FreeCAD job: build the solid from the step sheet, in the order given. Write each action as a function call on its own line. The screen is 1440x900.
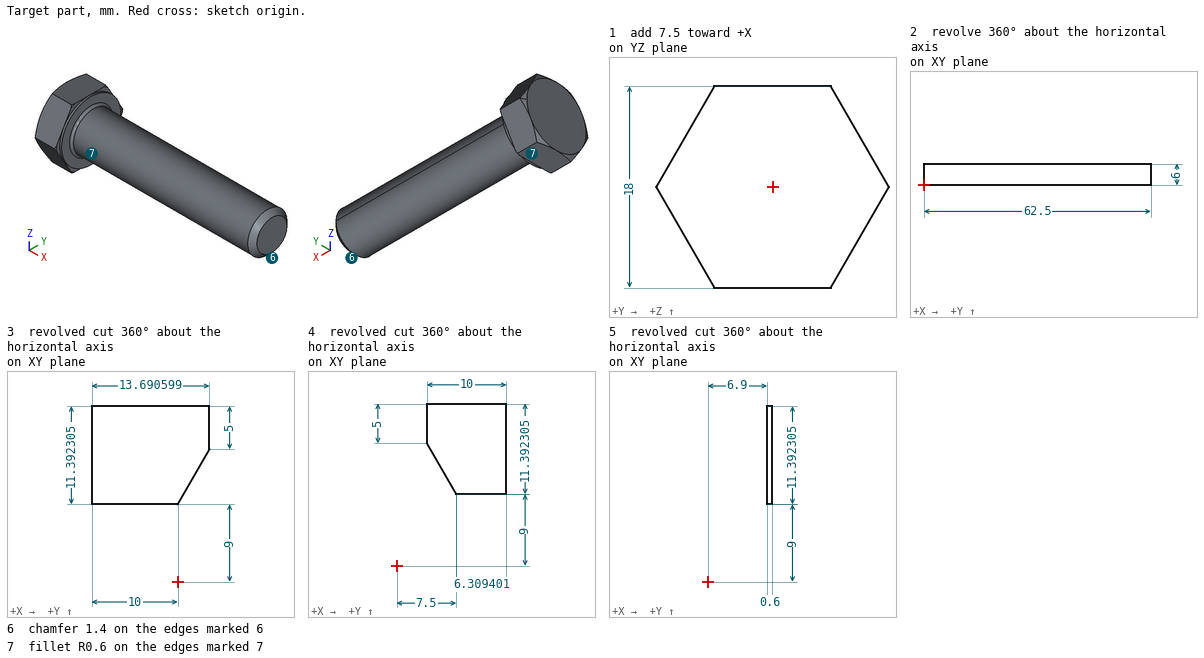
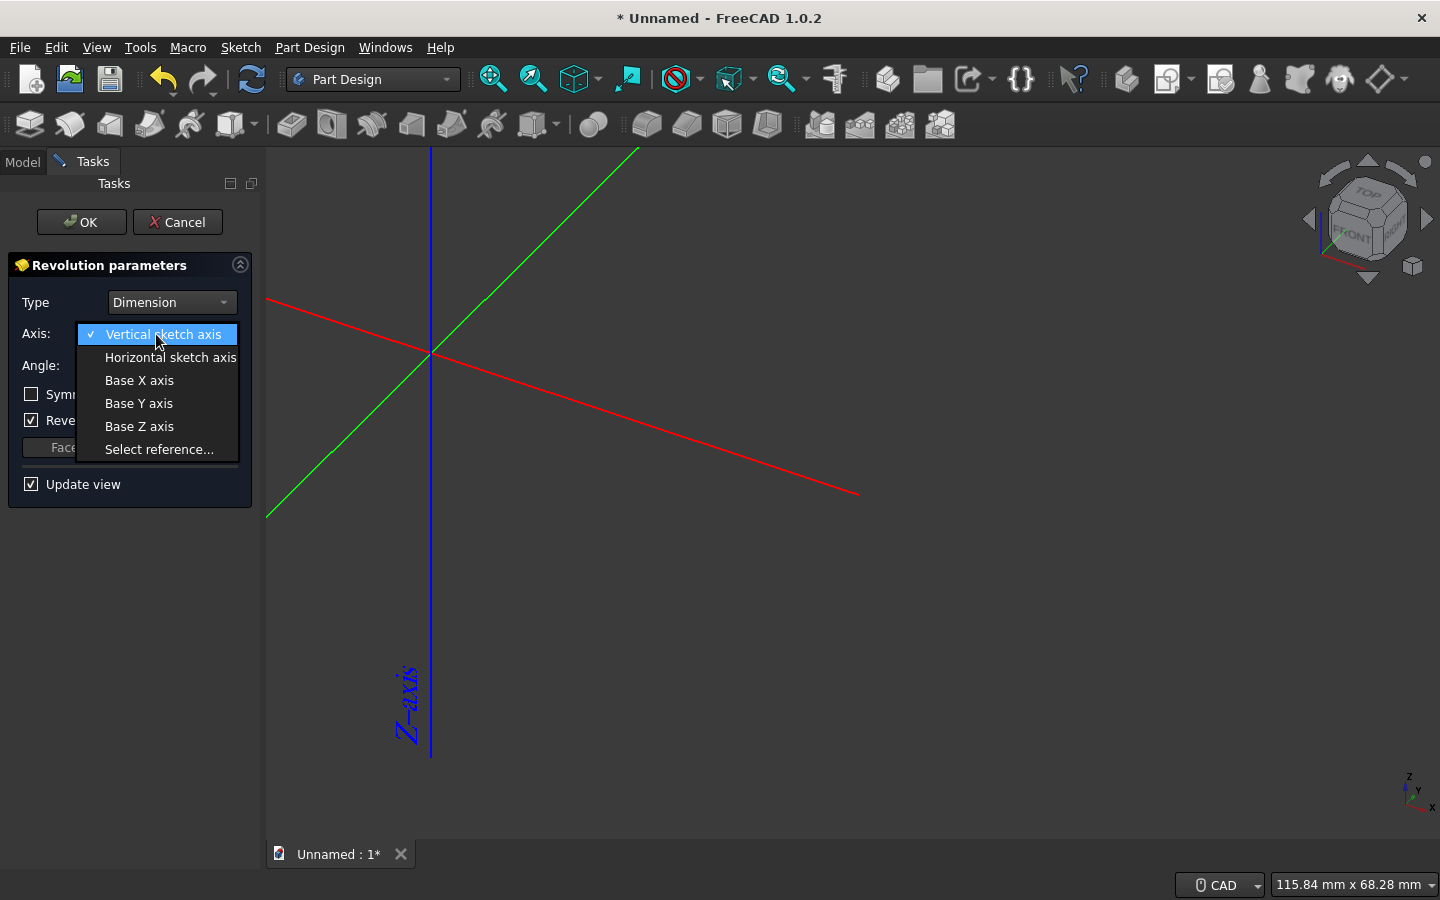
click(156, 358)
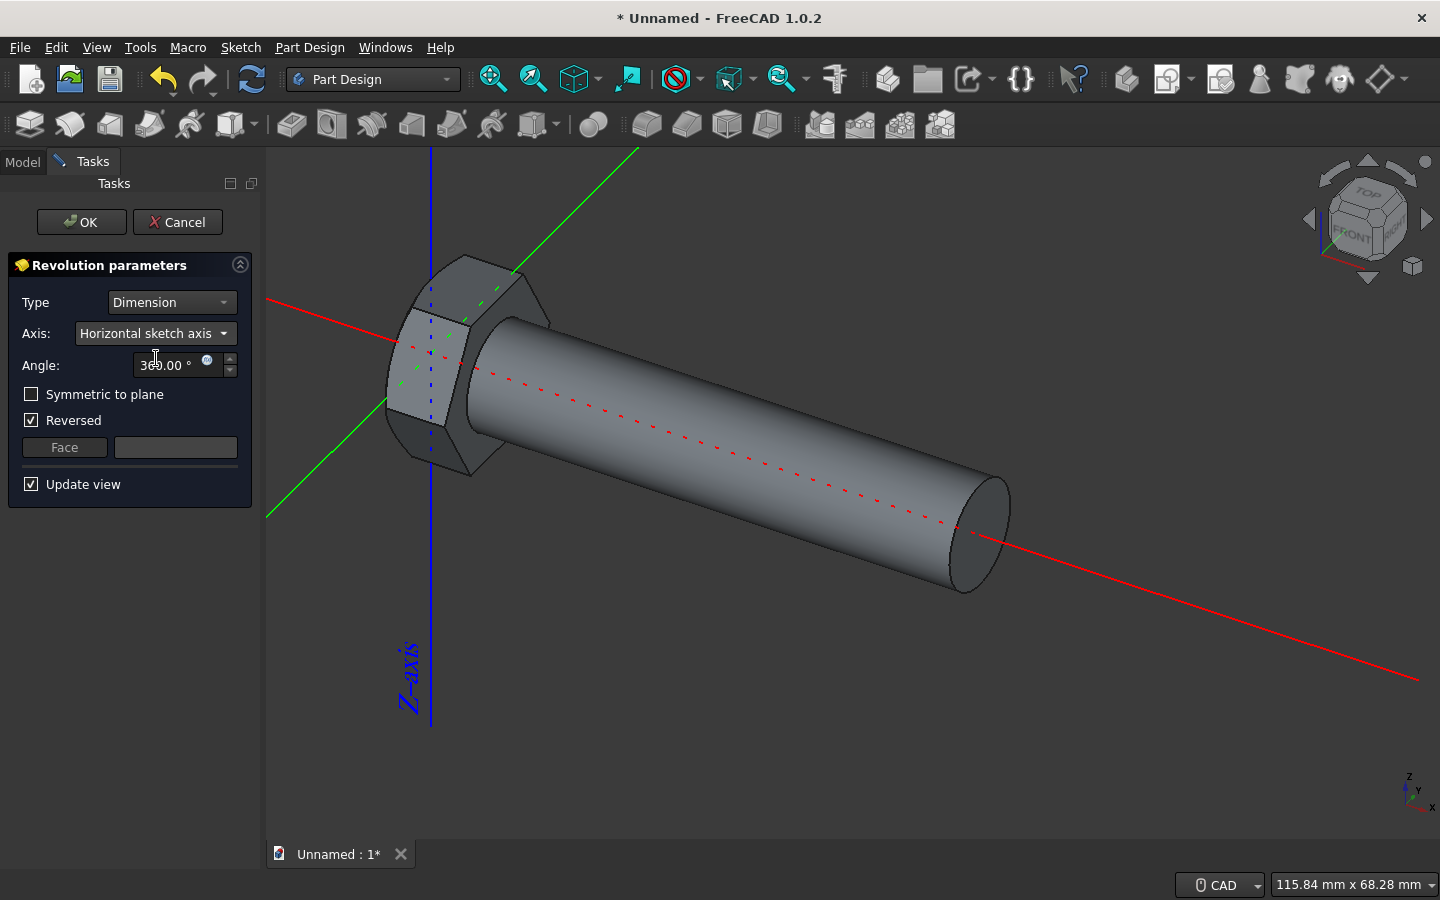
click(82, 222)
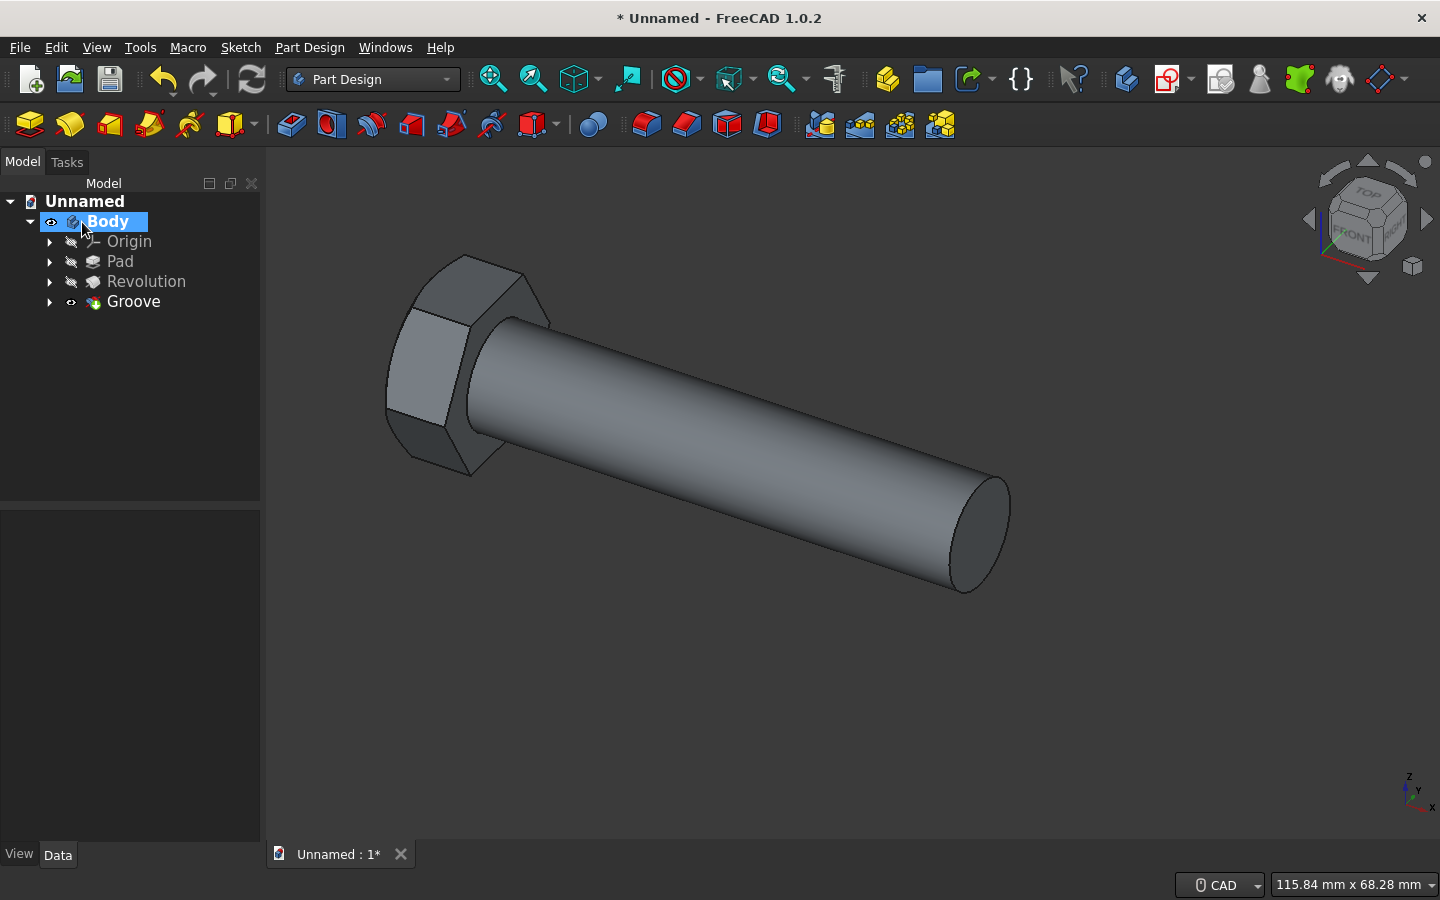
click(1168, 80)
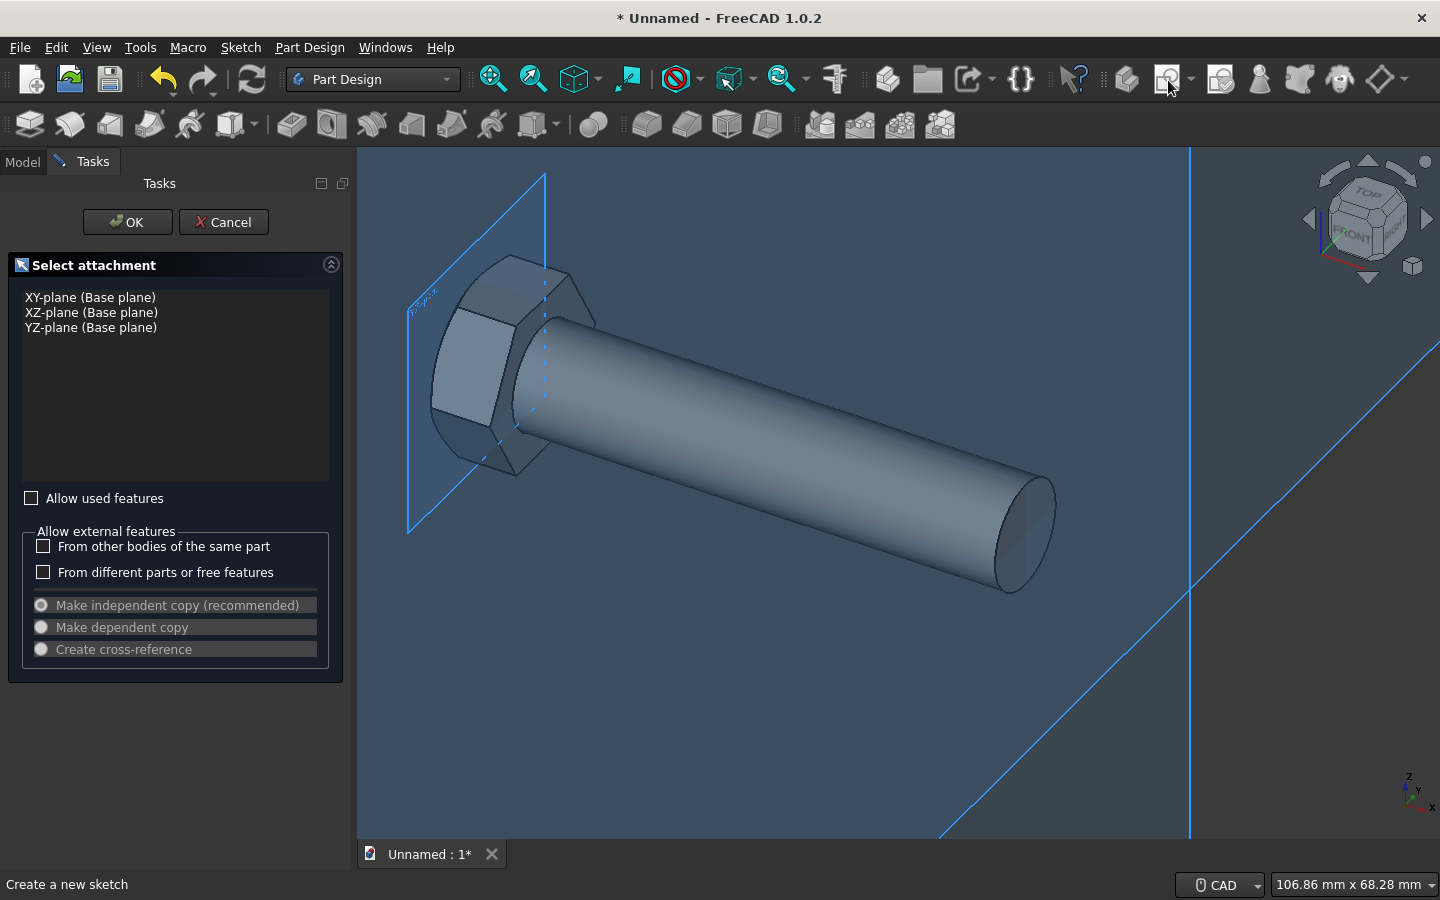
click(82, 298)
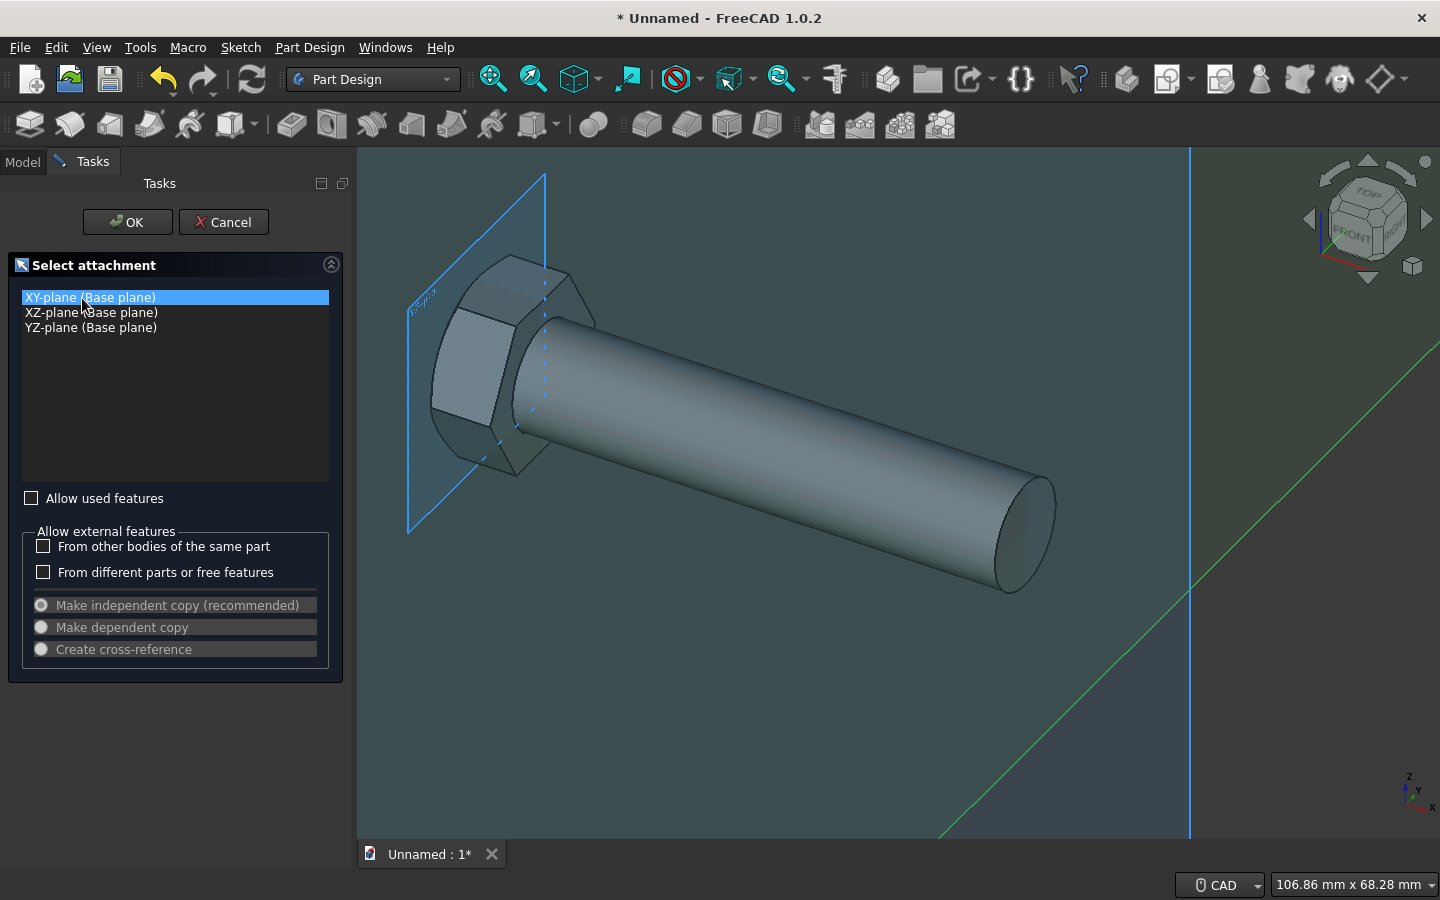
click(128, 222)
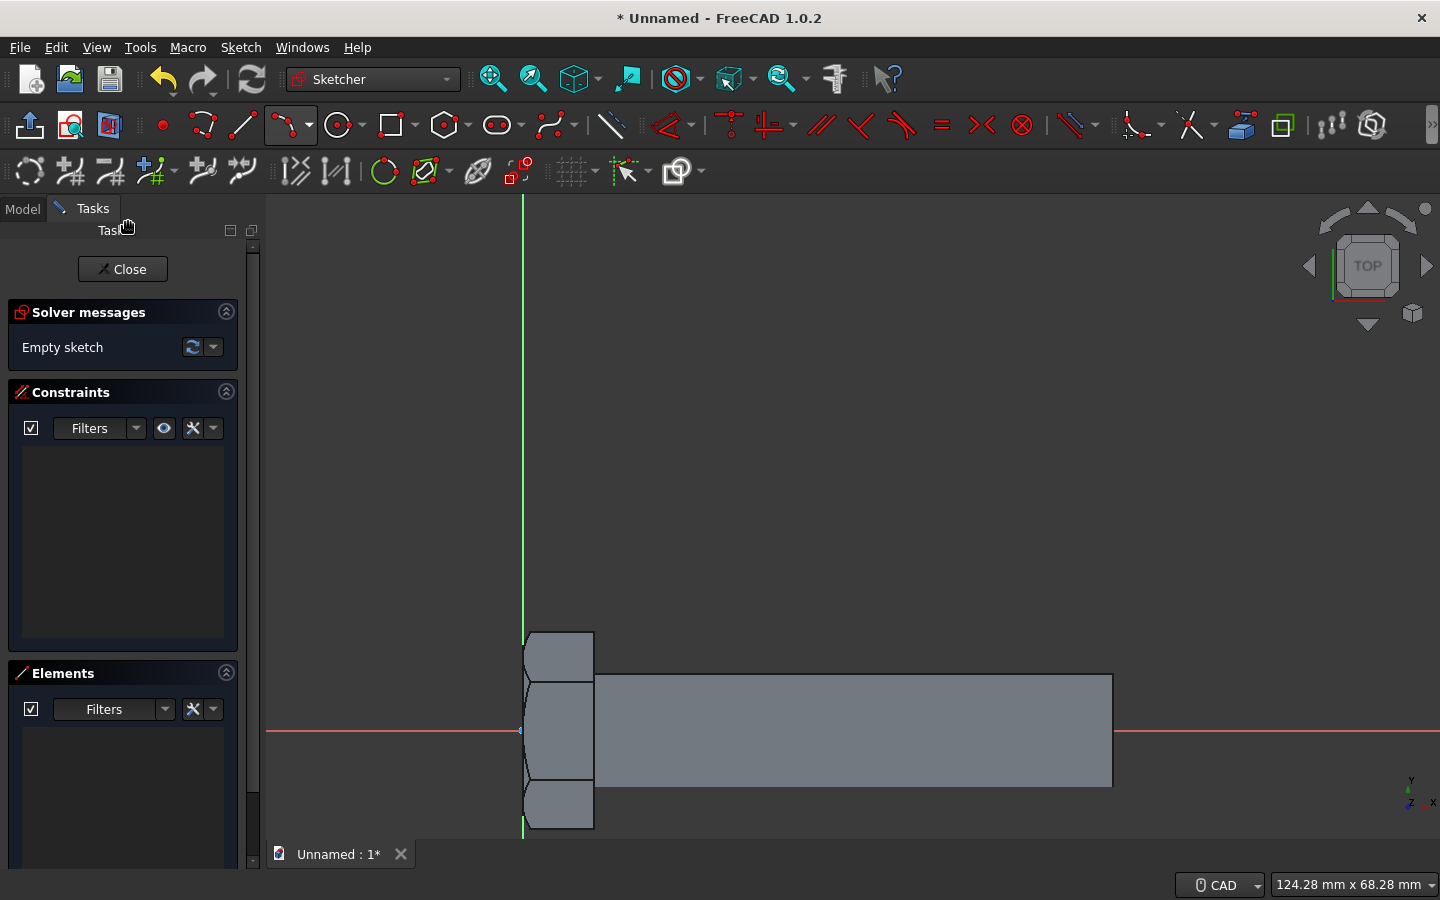
key(q)
key(s)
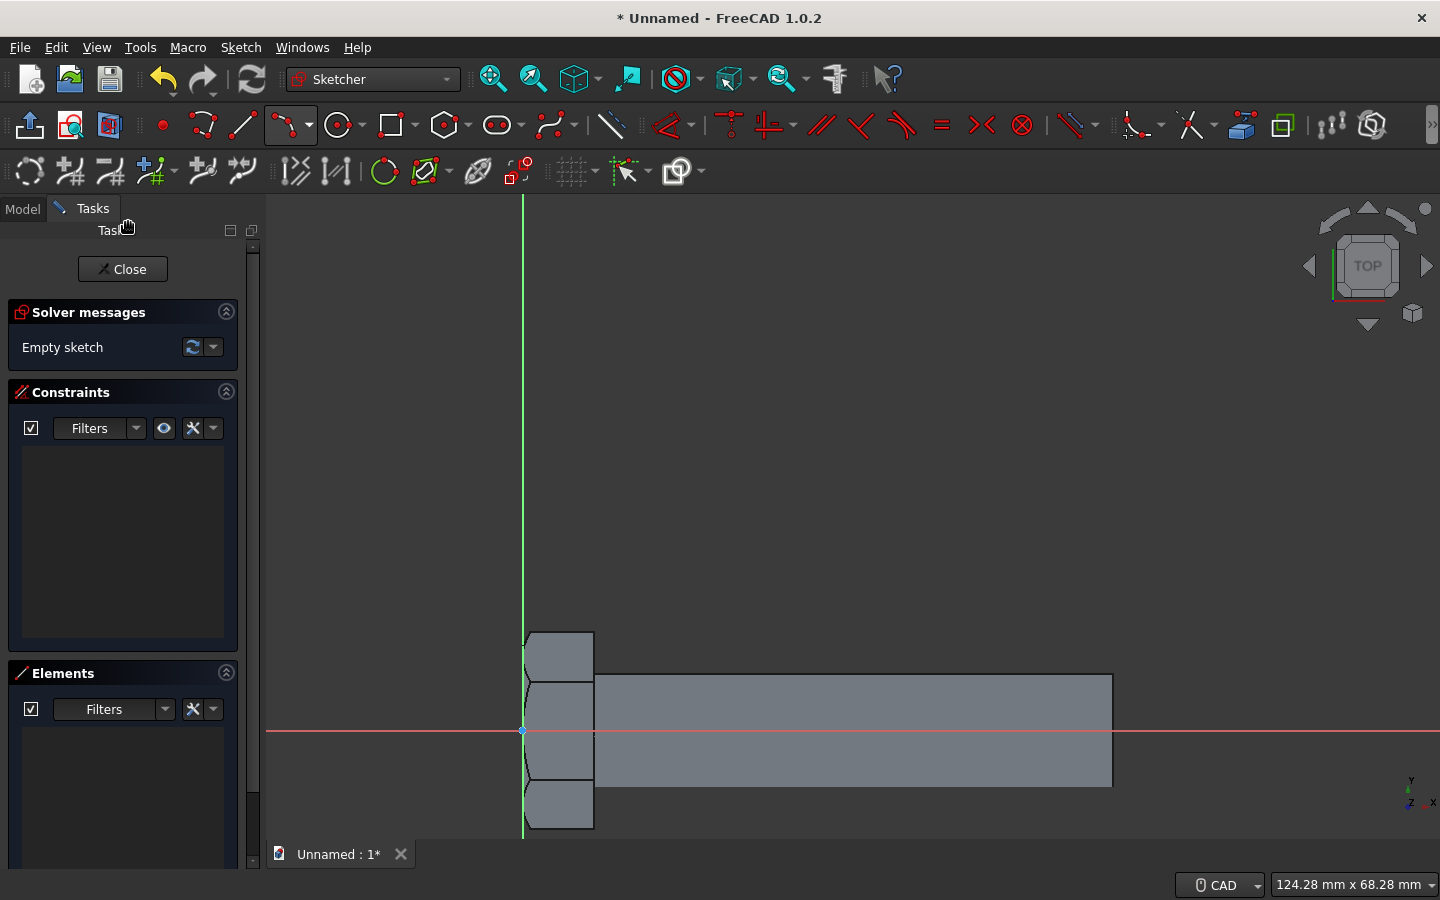
scroll(428, 730, up, 4)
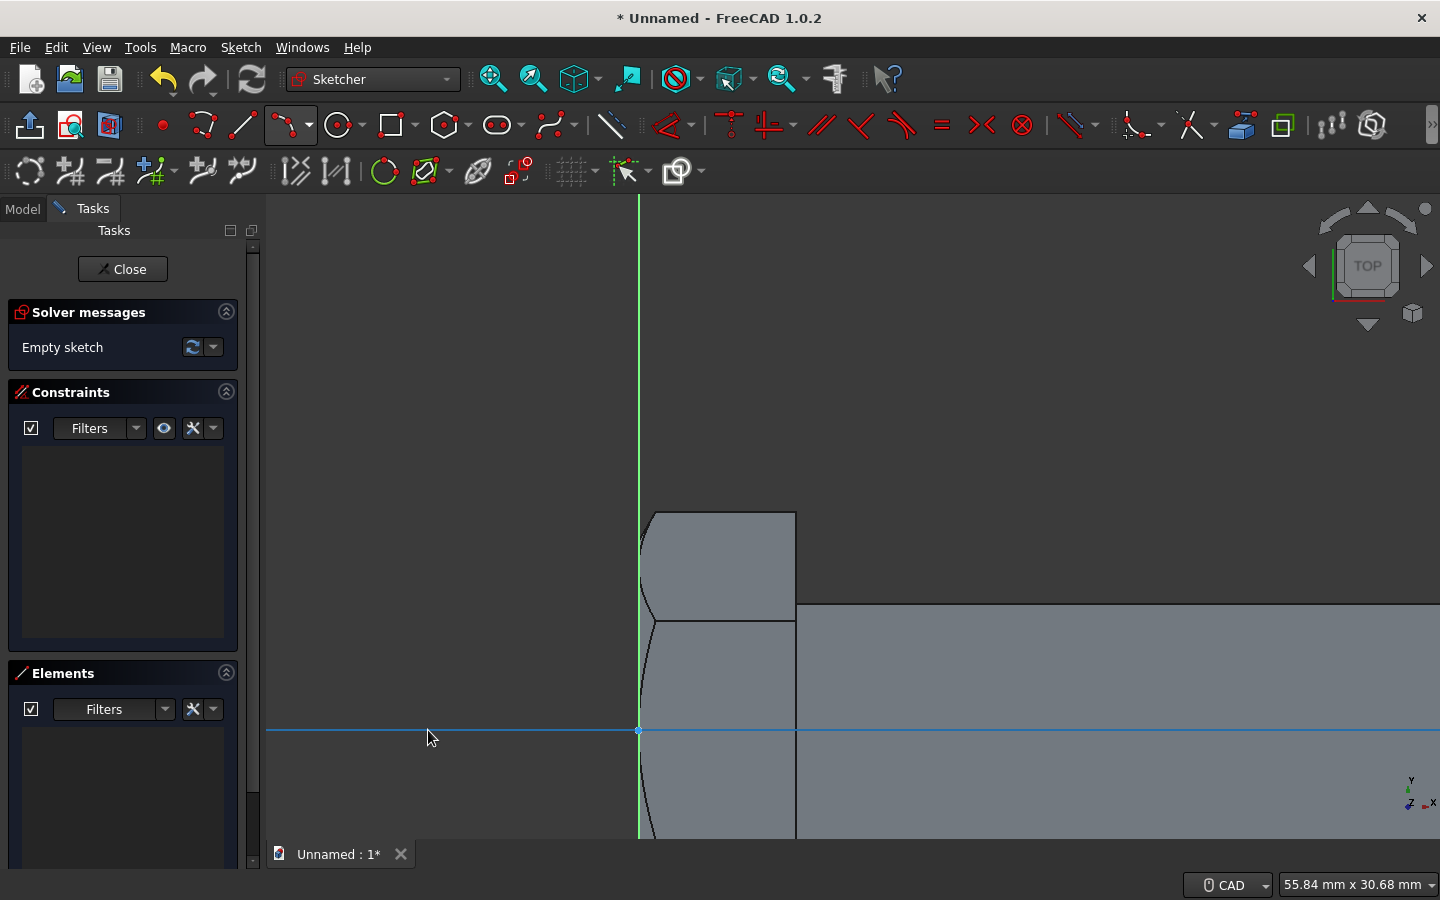
click(204, 126)